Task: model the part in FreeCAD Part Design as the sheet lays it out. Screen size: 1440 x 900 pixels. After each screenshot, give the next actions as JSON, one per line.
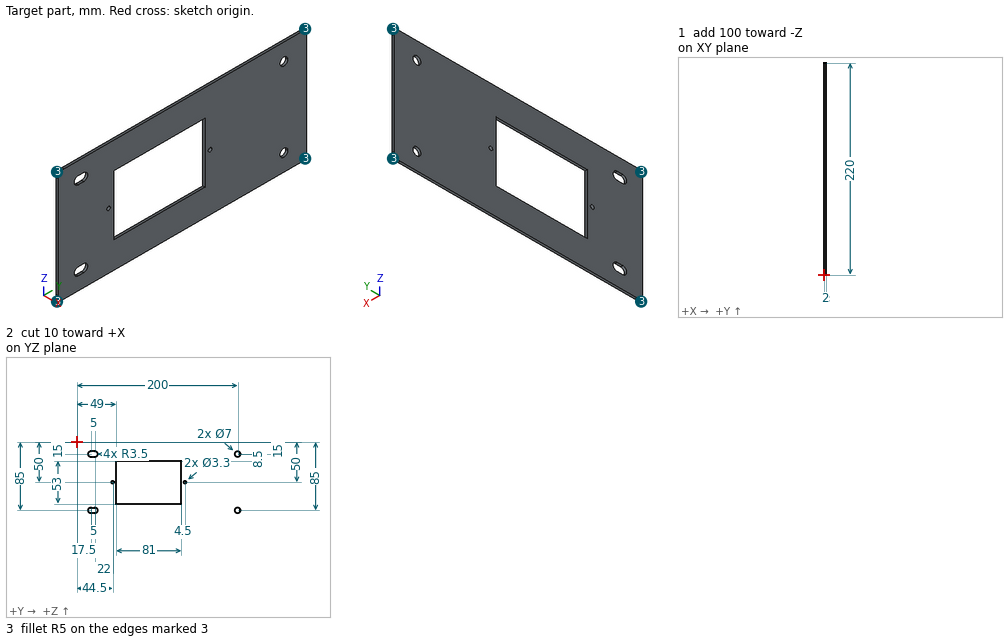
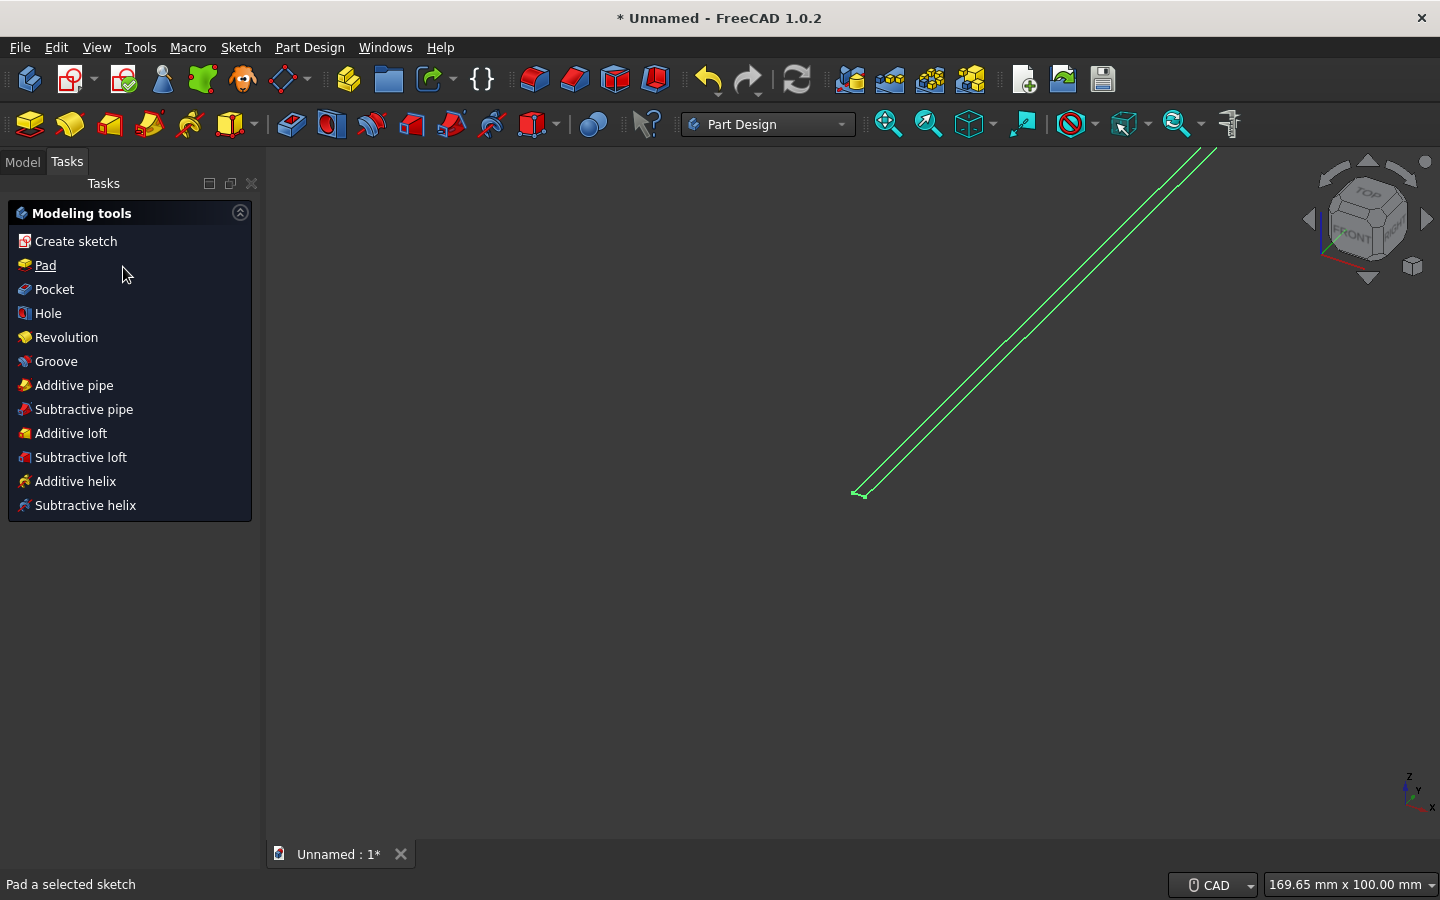
{"action": "left_click", "coordinate": [30, 124]}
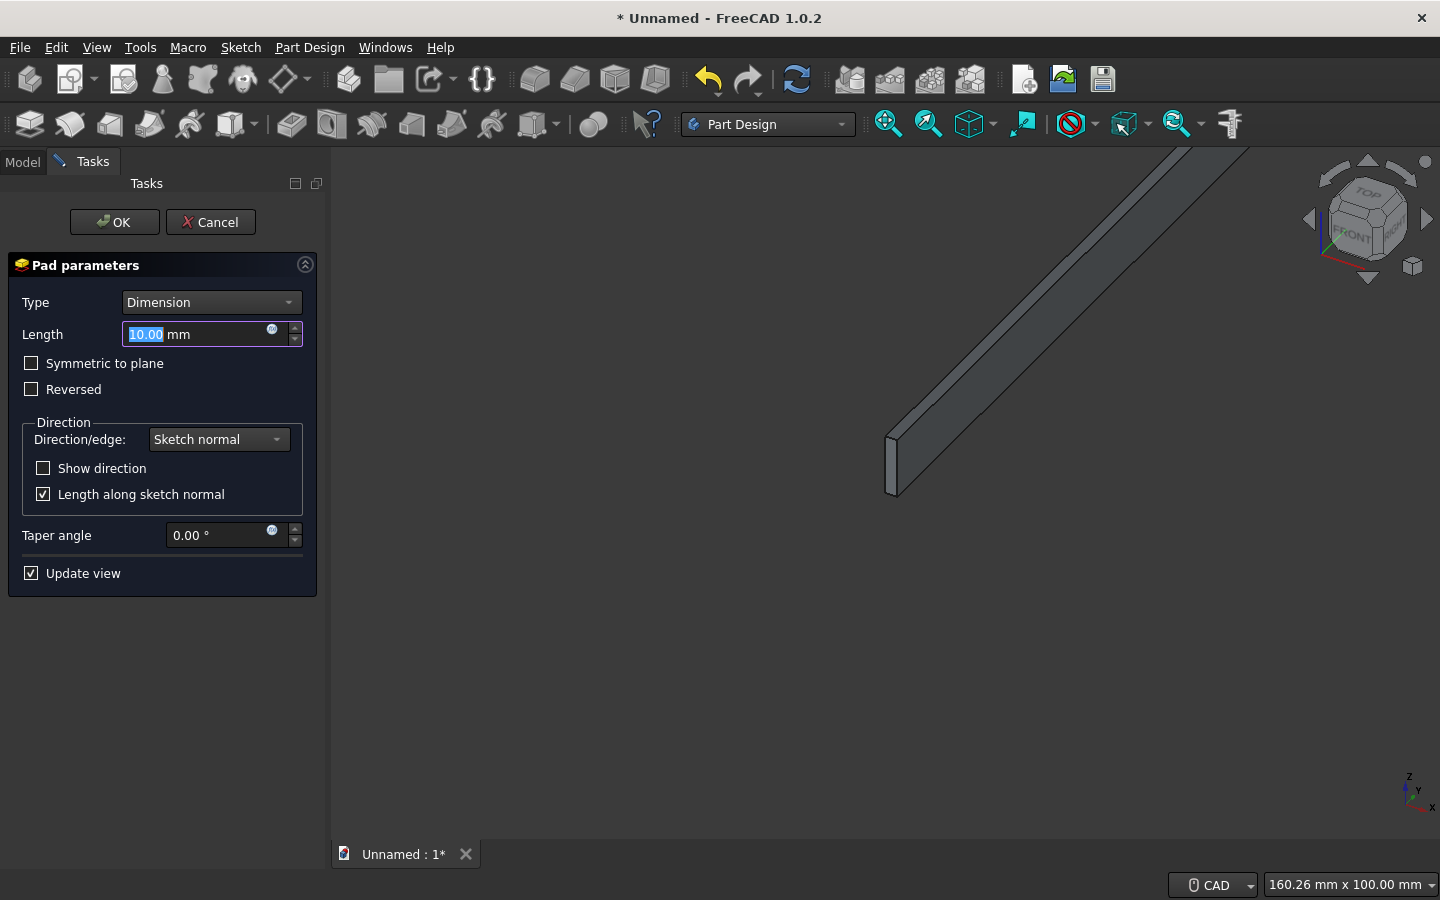
{"action": "type", "text": "100"}
{"action": "key", "text": "Tab"}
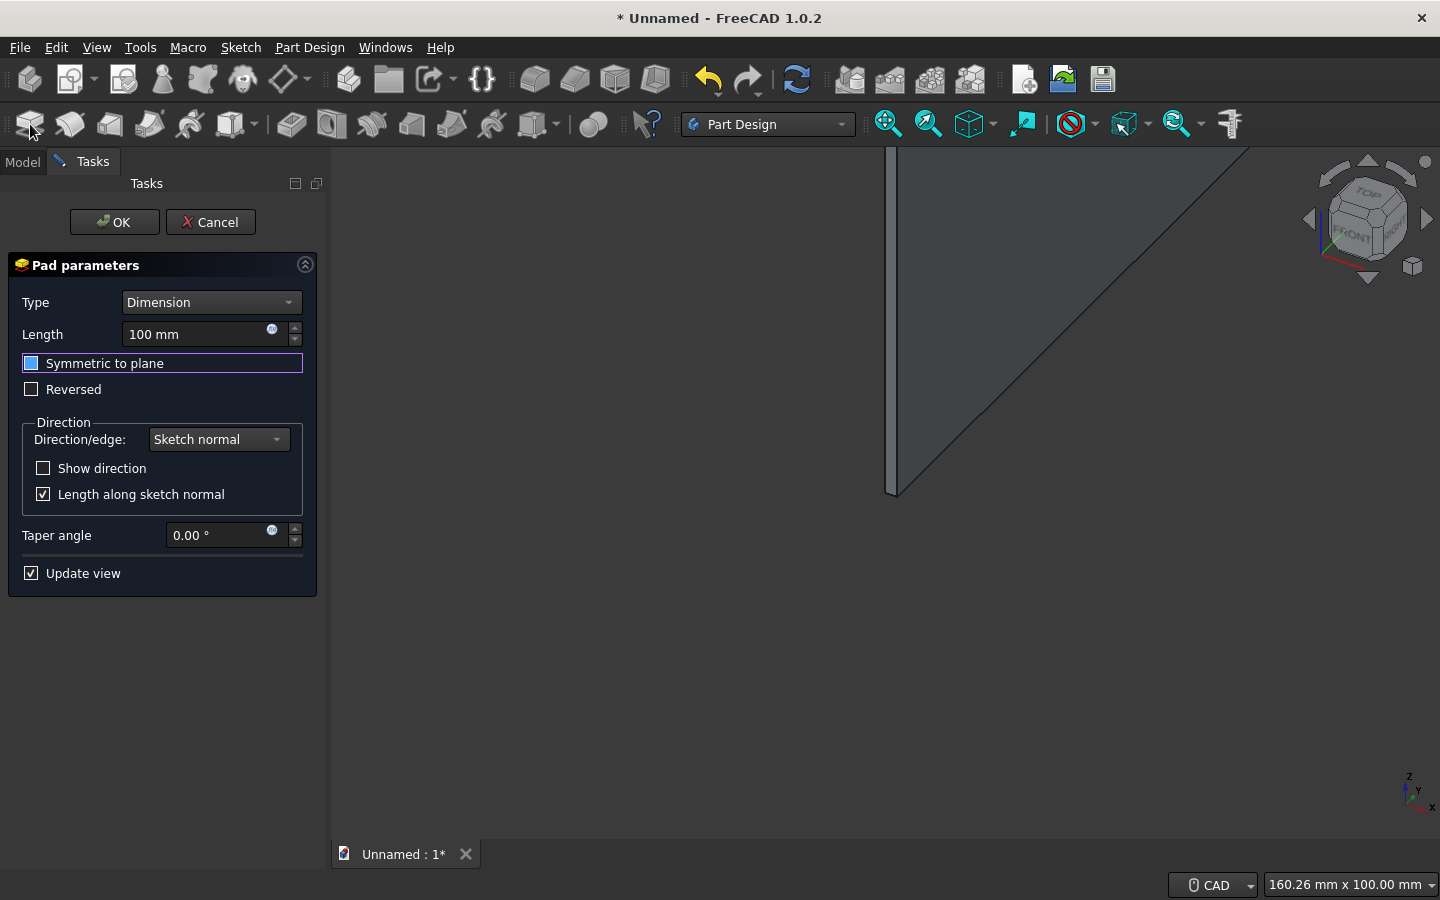
{"action": "left_click", "coordinate": [30, 389]}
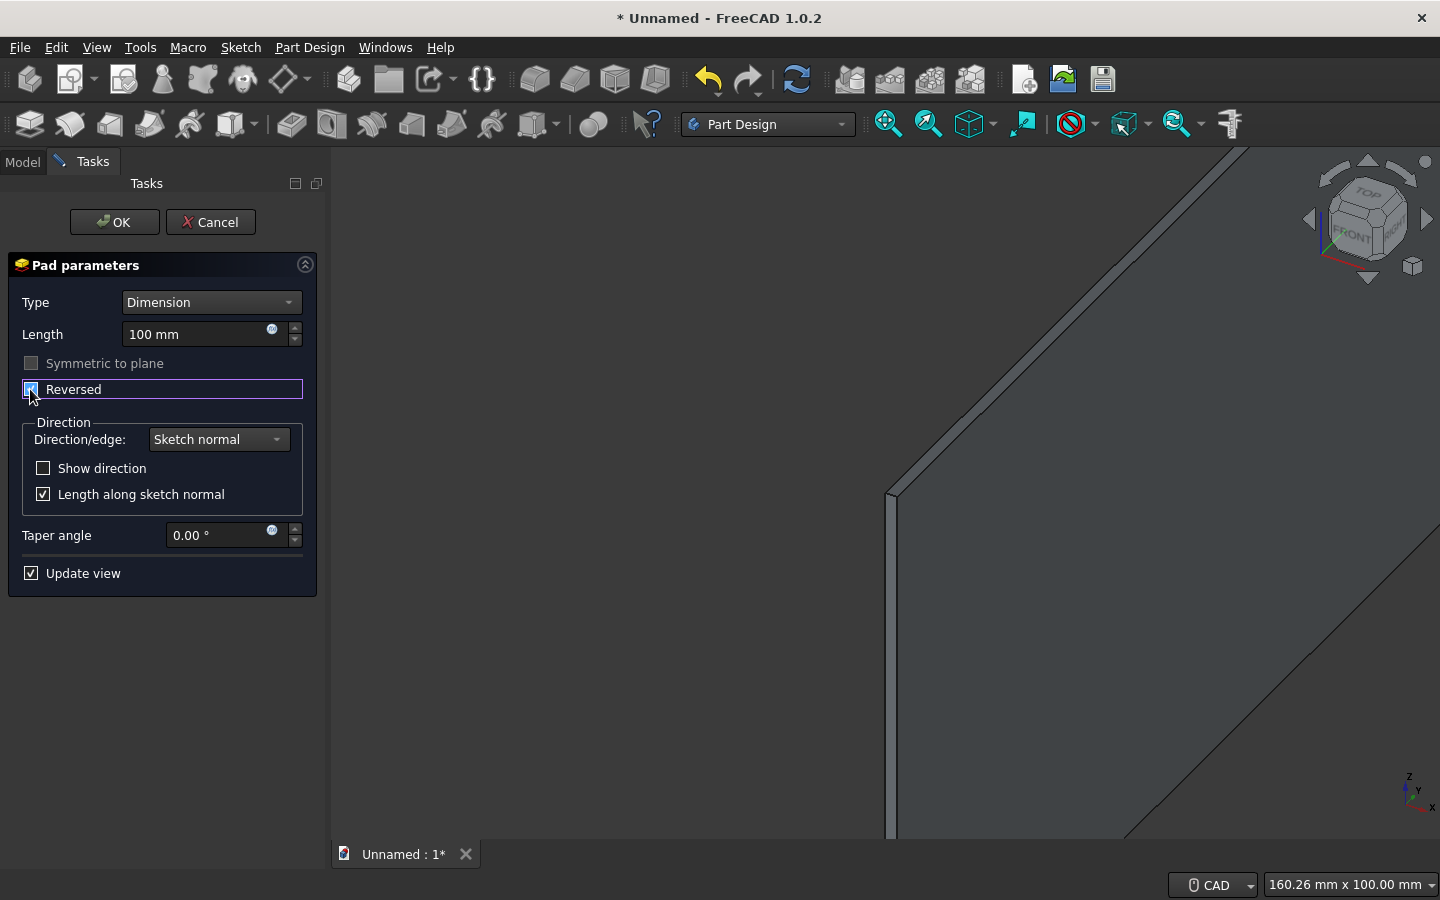
{"action": "left_click", "coordinate": [115, 222]}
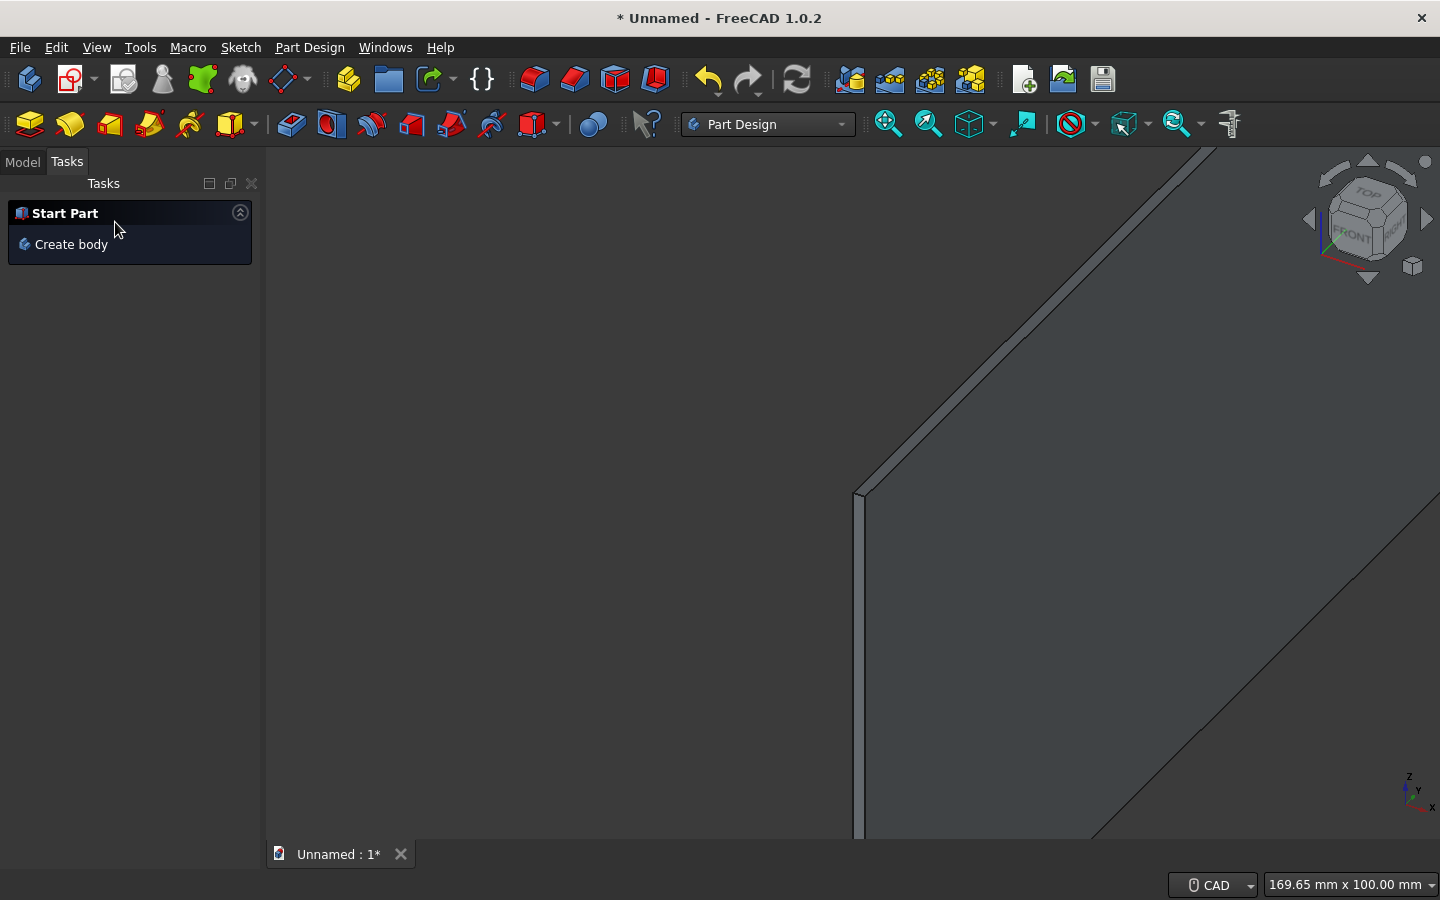
{"action": "left_click", "coordinate": [890, 124]}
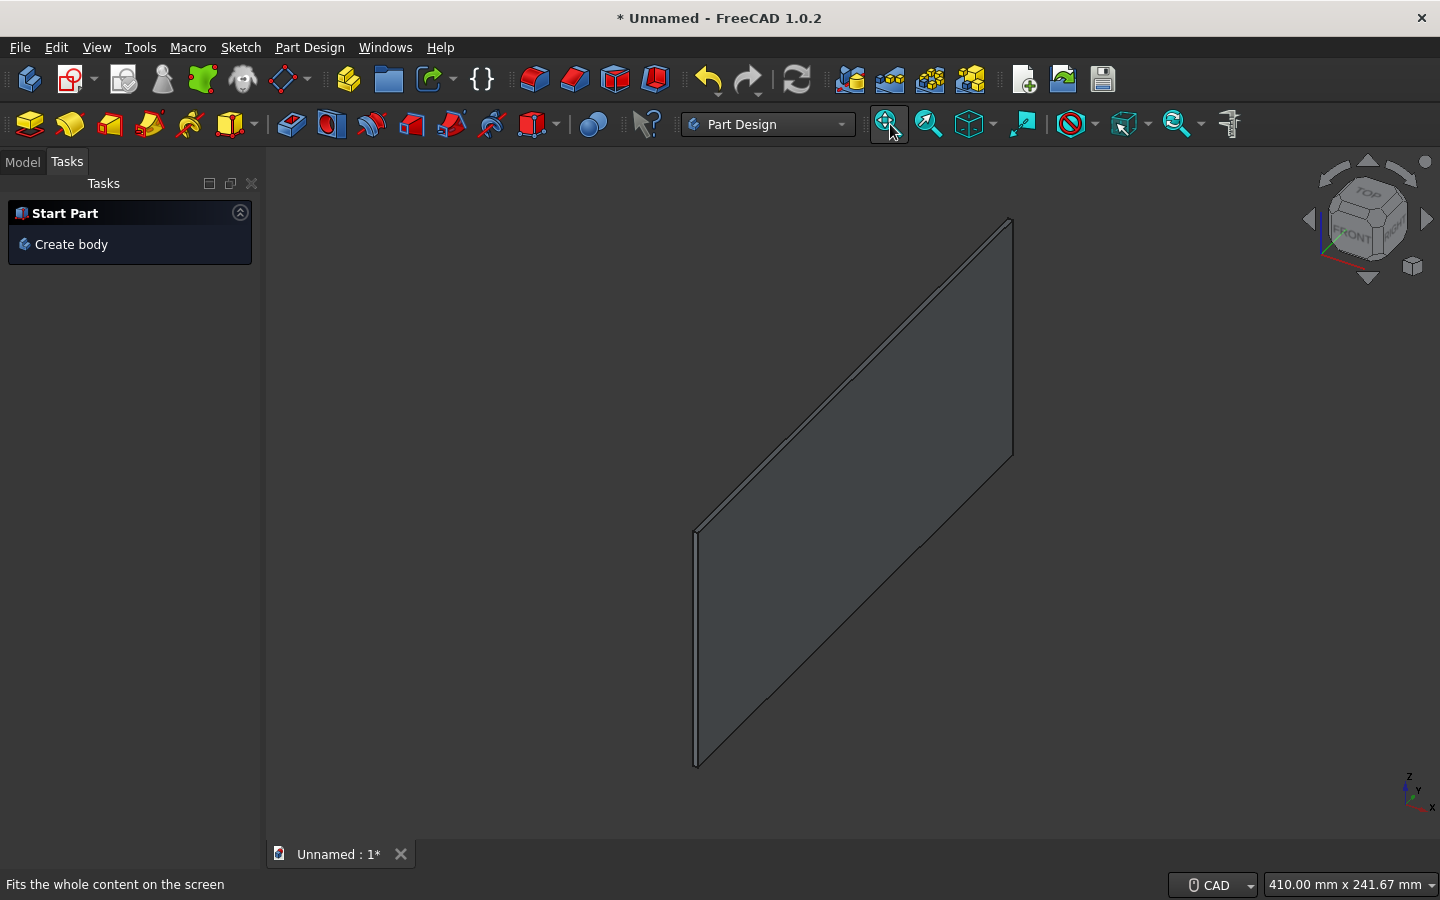
{"action": "left_click", "coordinate": [70, 80]}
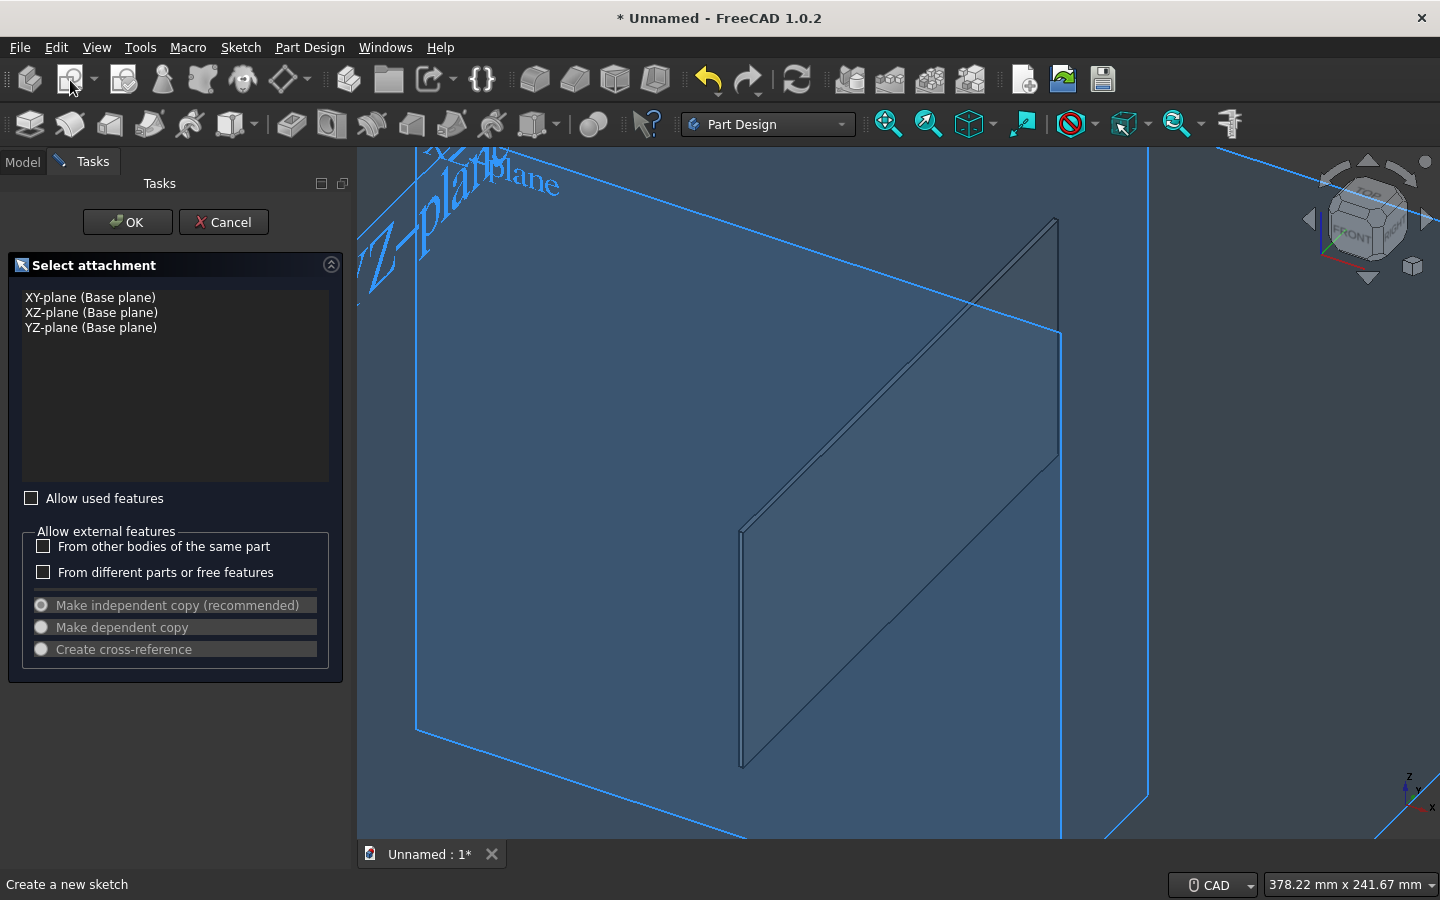
{"action": "left_click", "coordinate": [82, 328]}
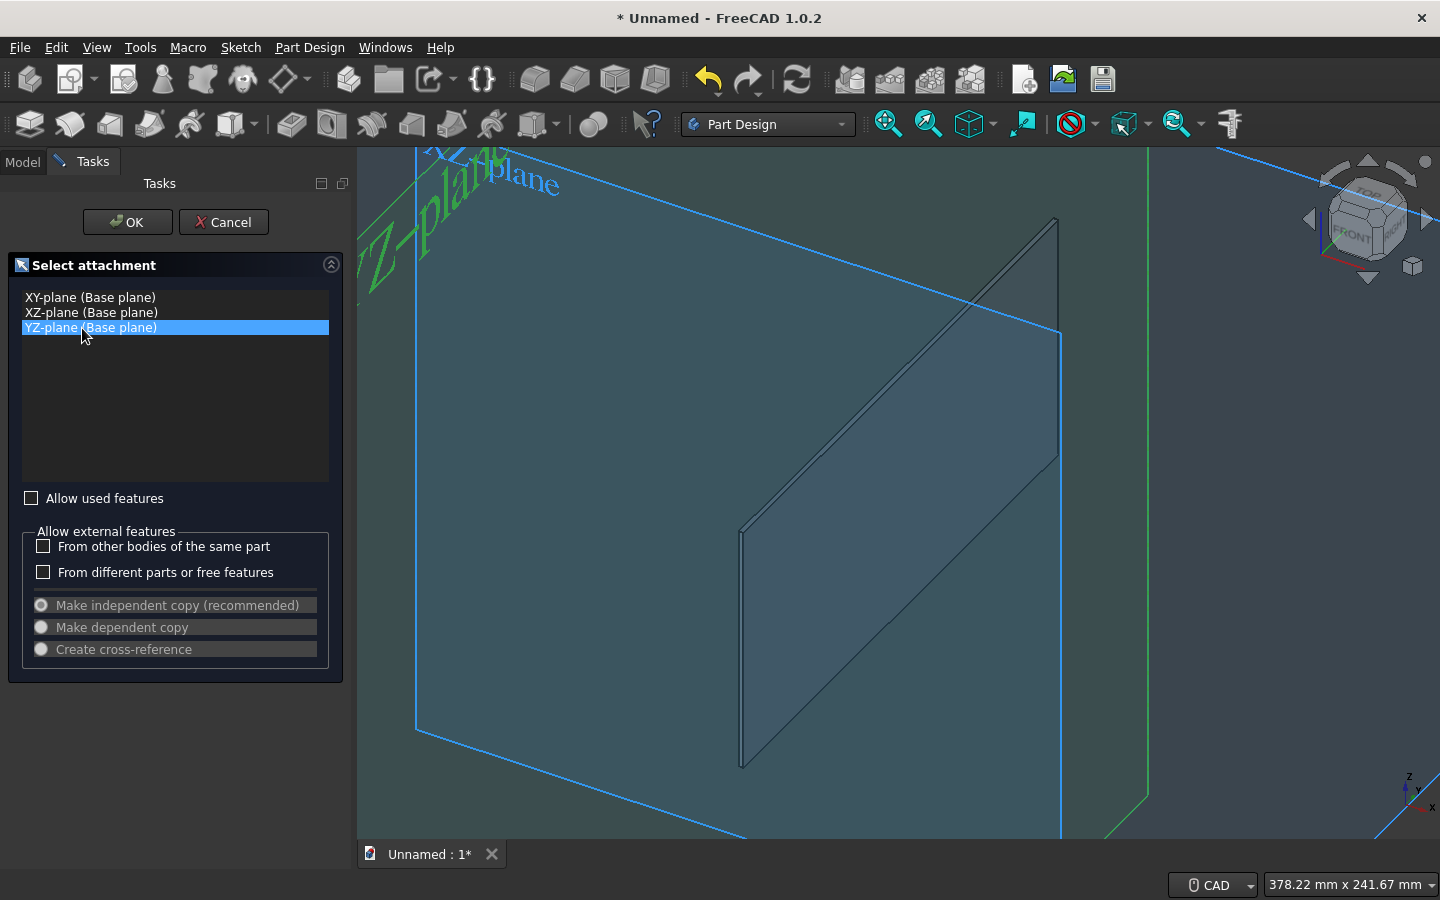
{"action": "left_click", "coordinate": [128, 222]}